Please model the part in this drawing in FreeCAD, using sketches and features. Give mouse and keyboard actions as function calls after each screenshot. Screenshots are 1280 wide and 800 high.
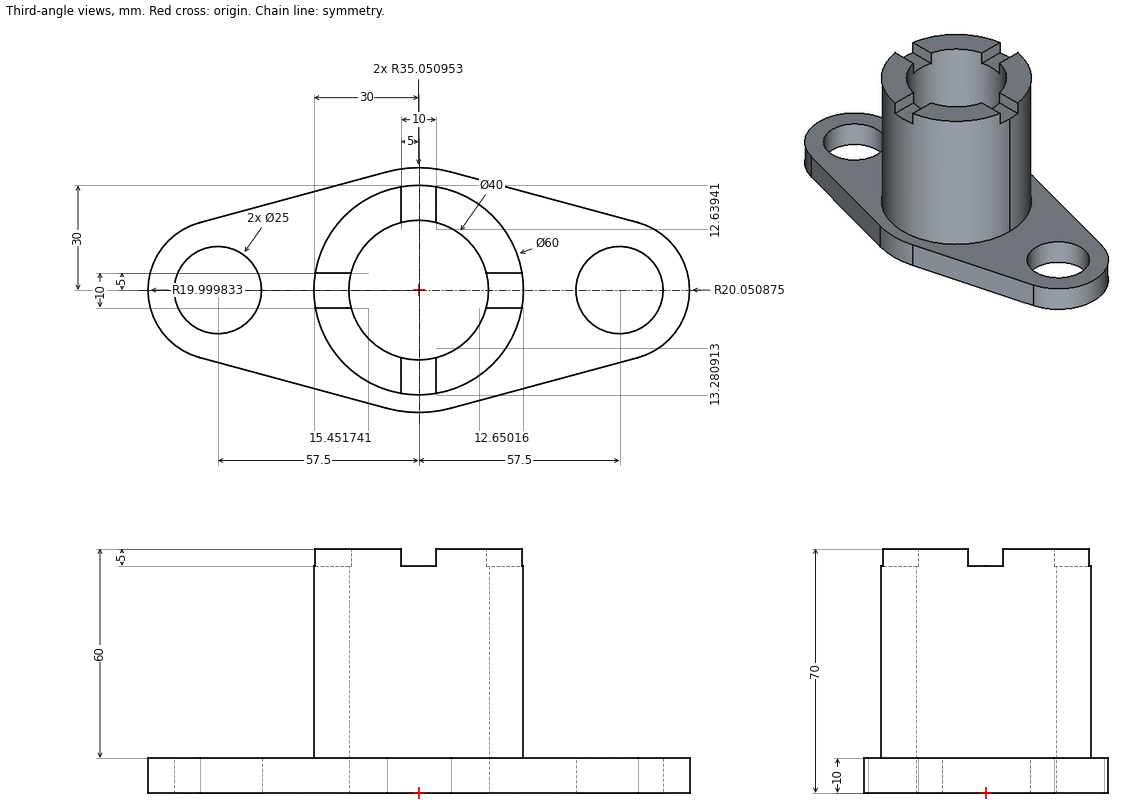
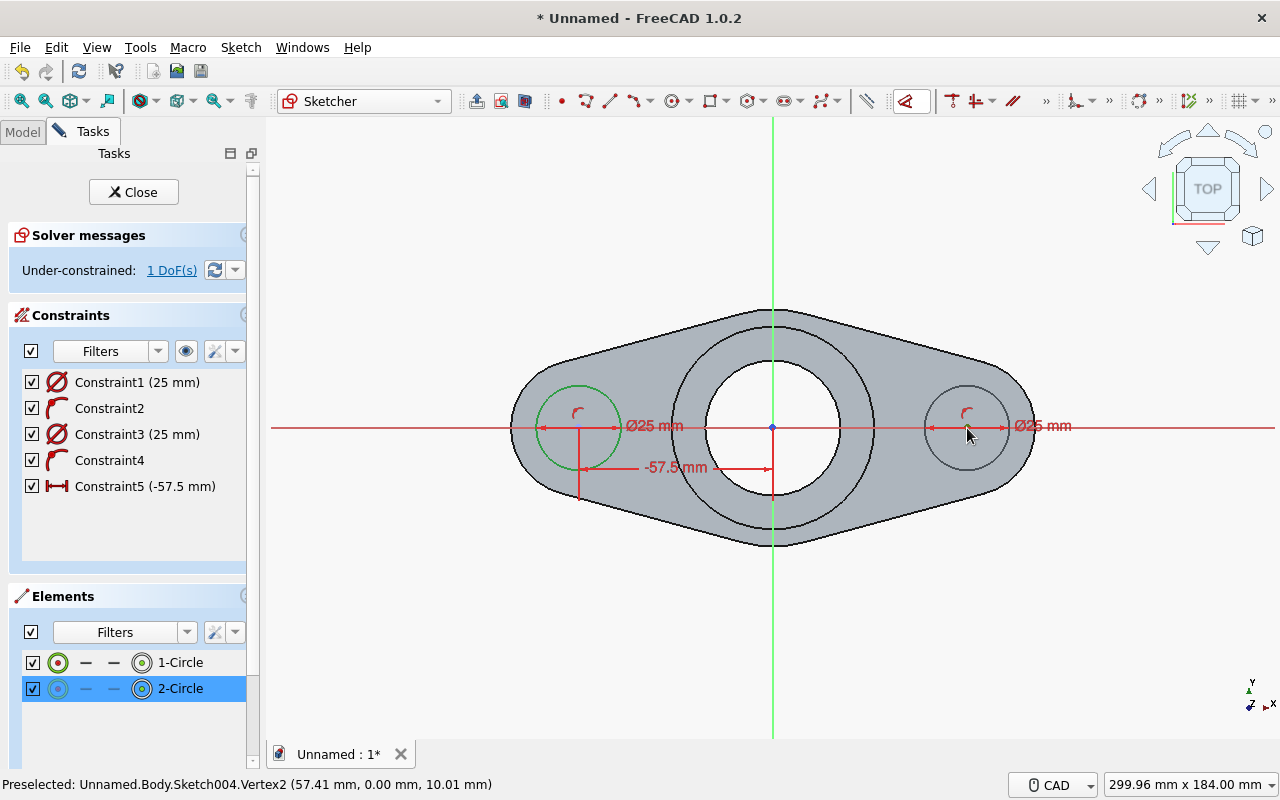
key(l)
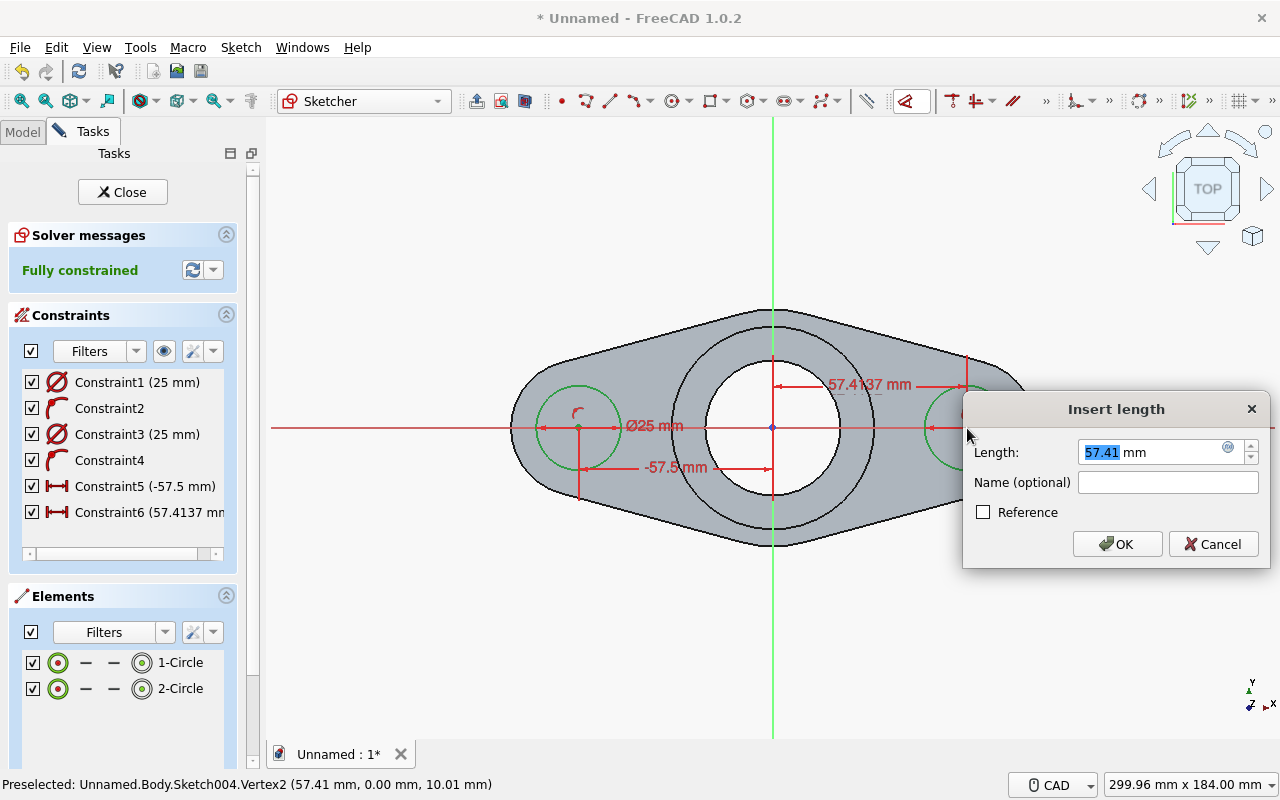
text(57.5)
key(Return)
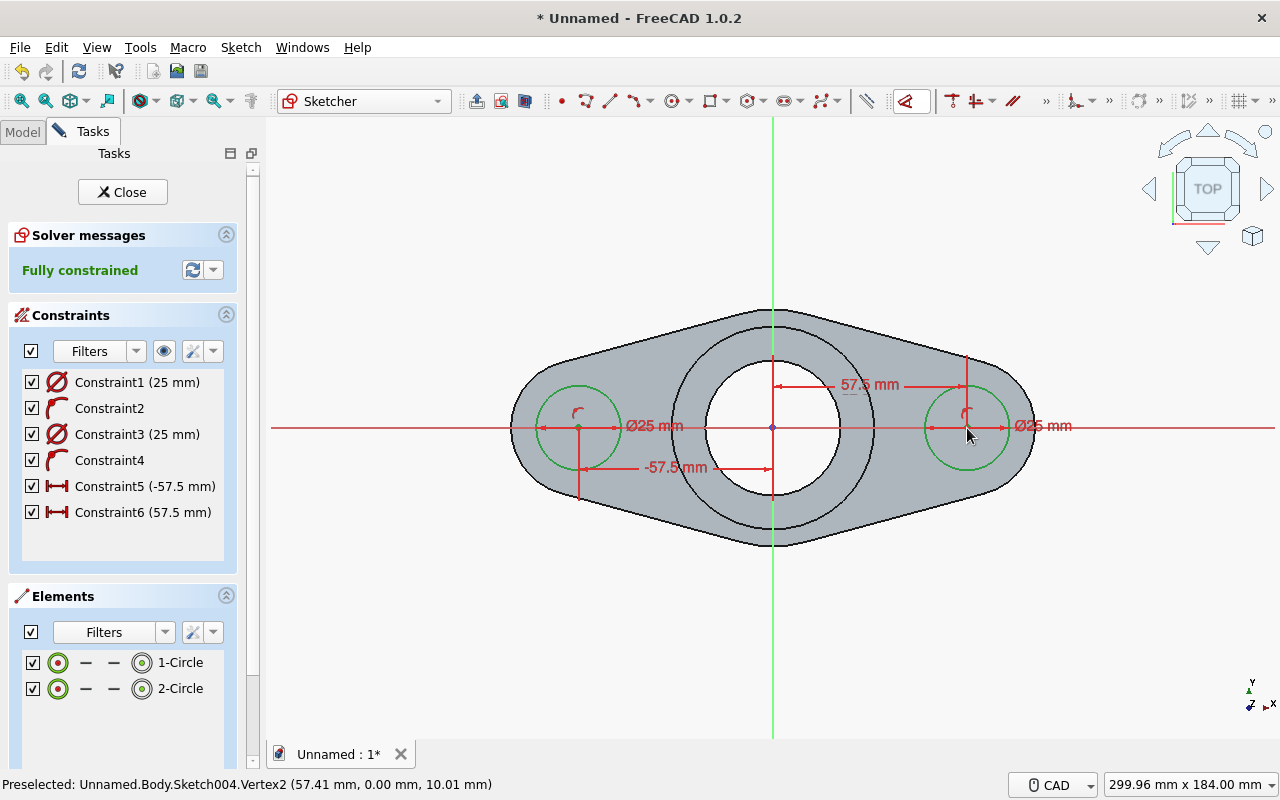
click(123, 192)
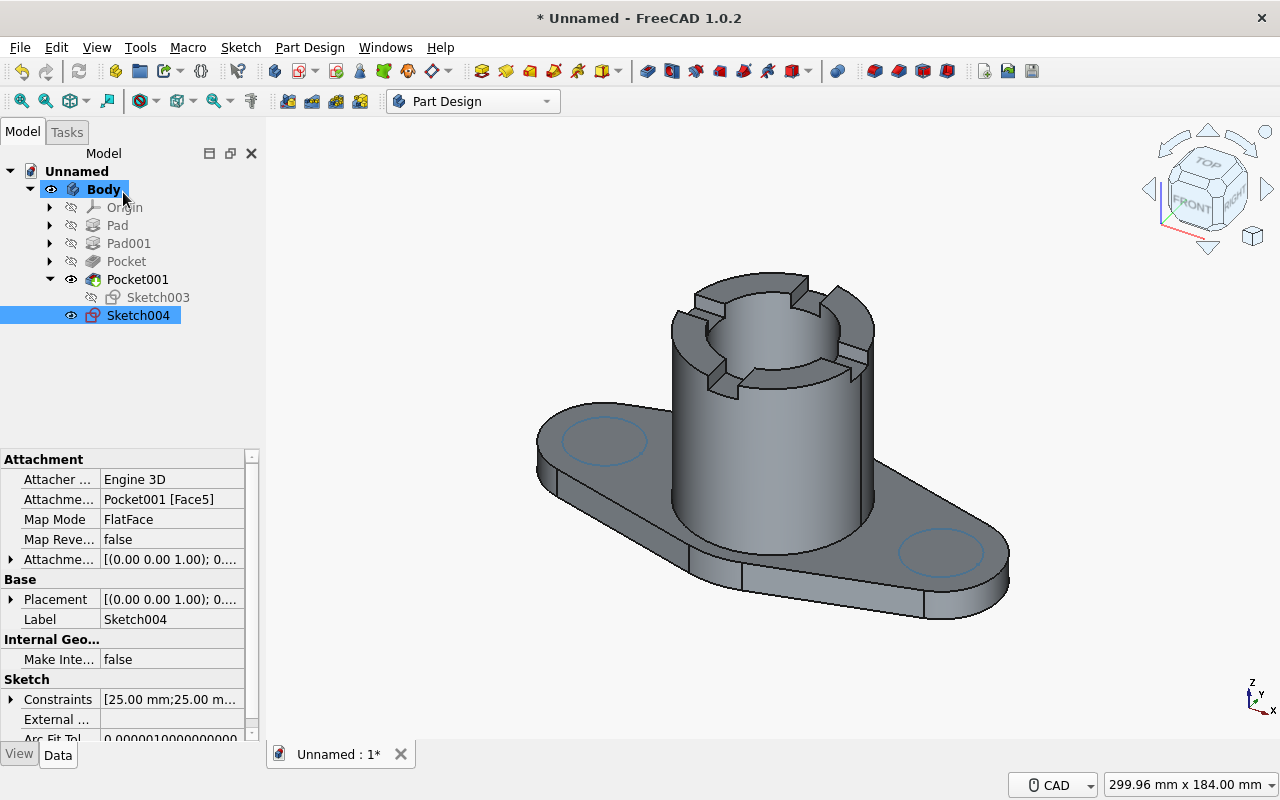
click(648, 72)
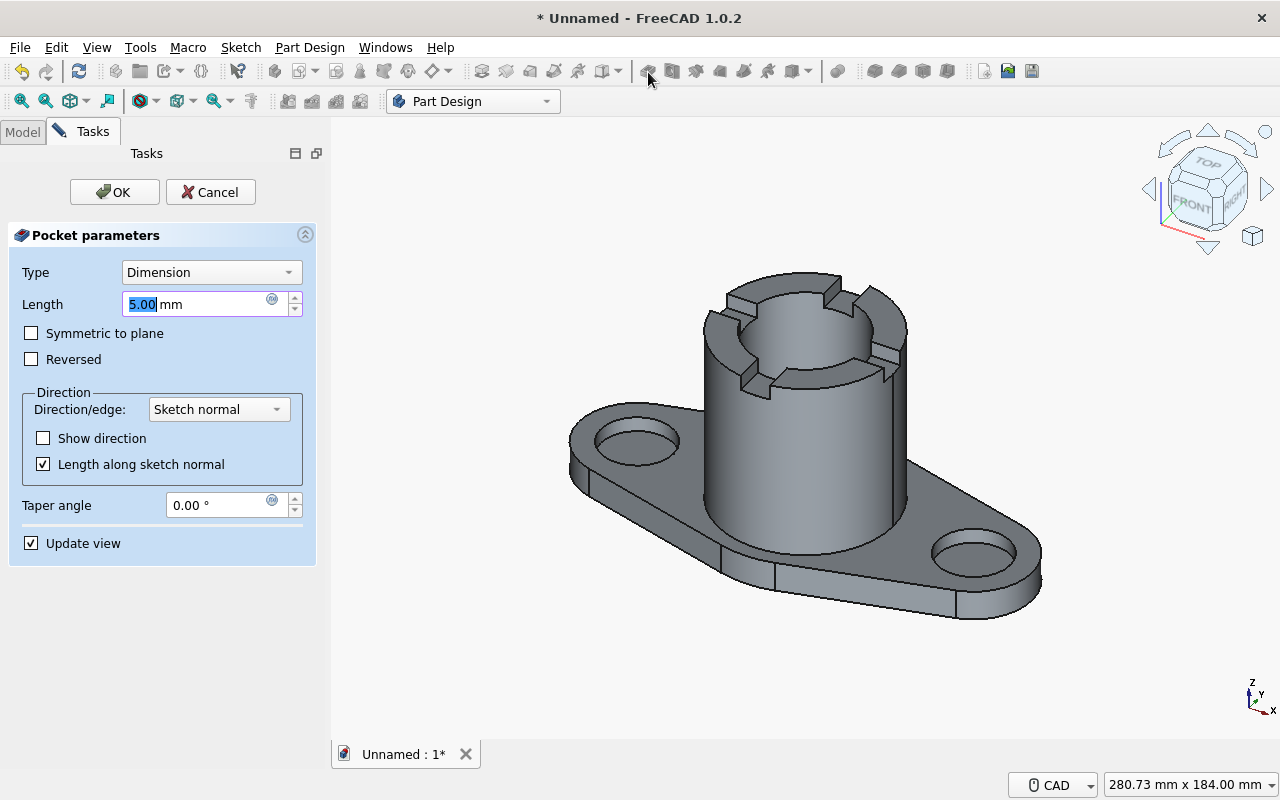
text(10)
key(Tab)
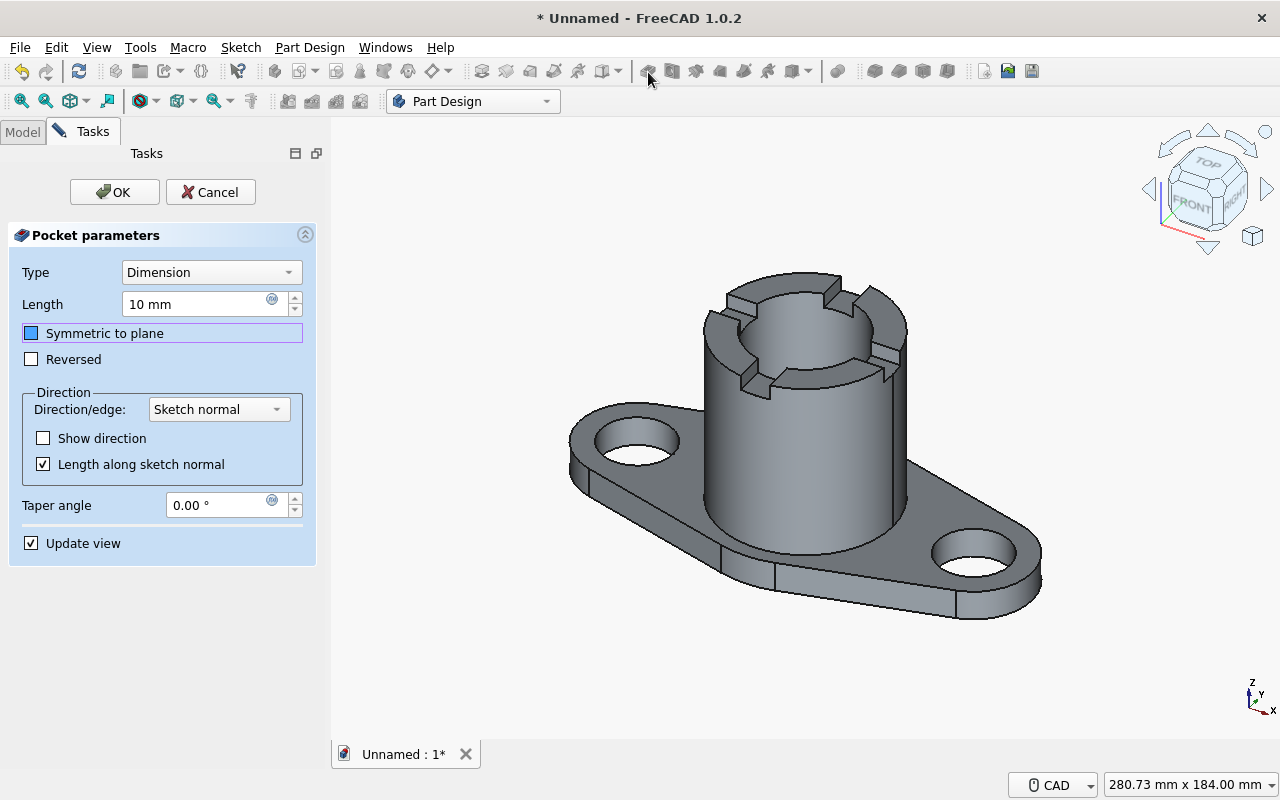
click(115, 192)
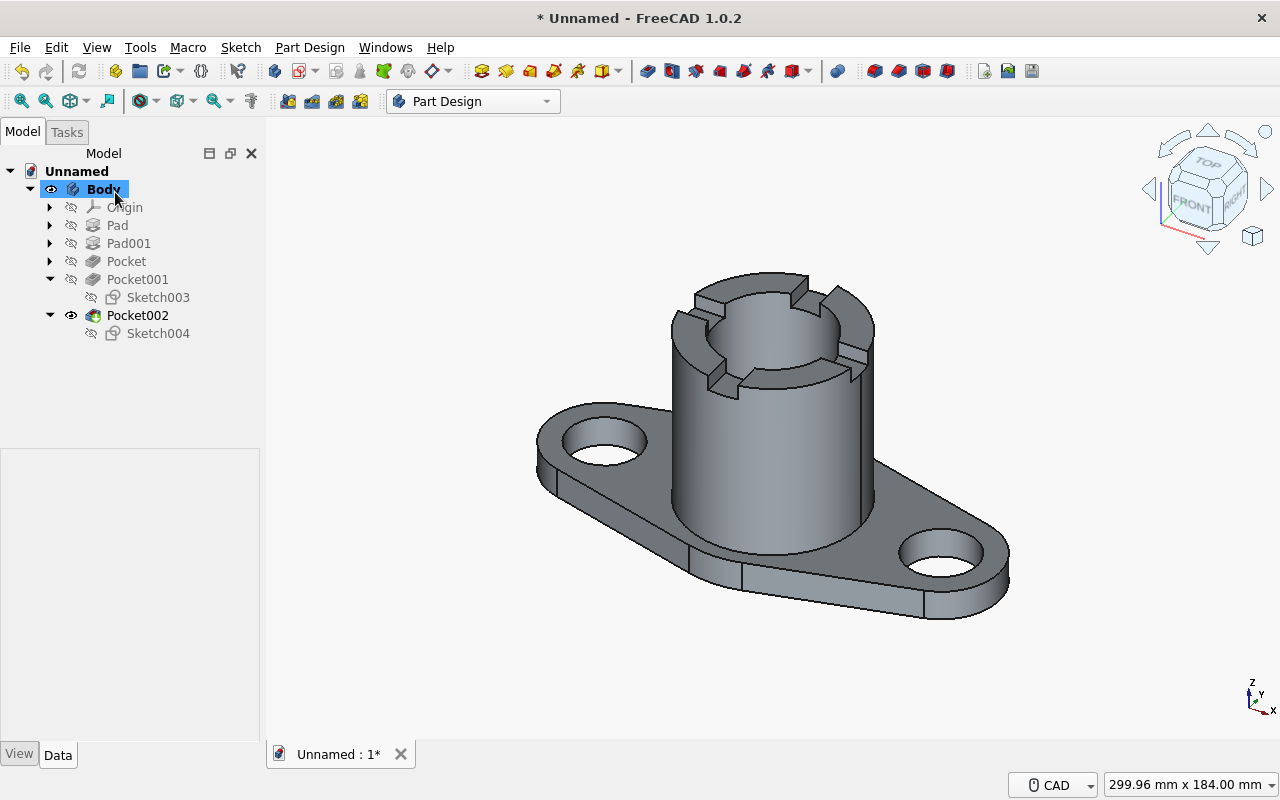
key(0)